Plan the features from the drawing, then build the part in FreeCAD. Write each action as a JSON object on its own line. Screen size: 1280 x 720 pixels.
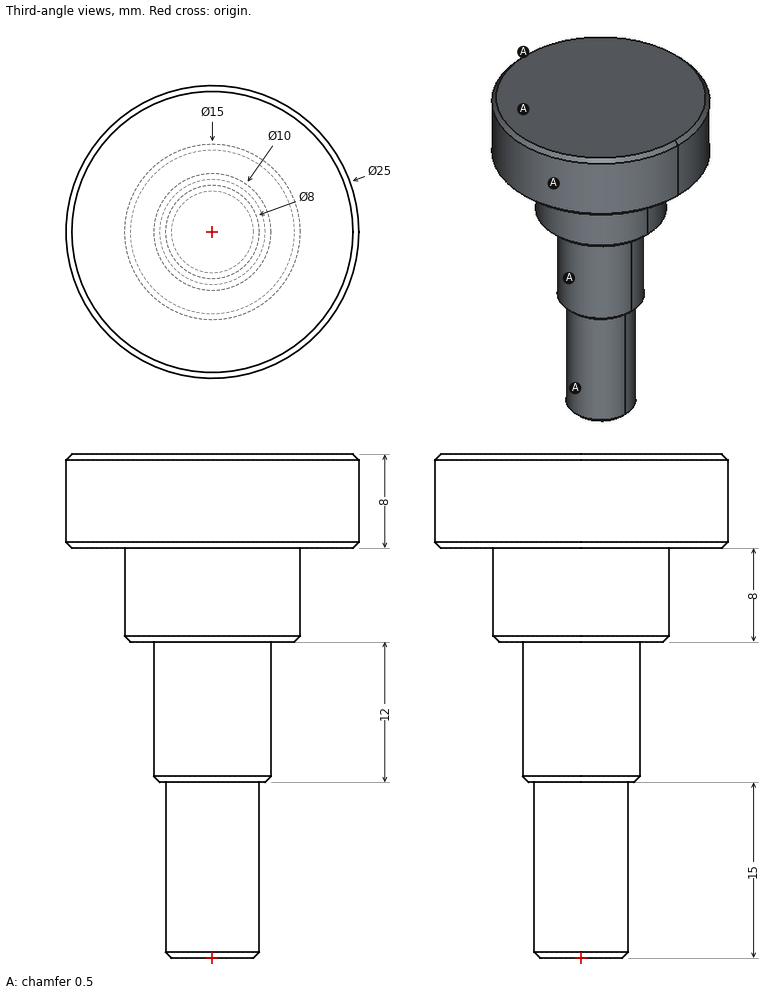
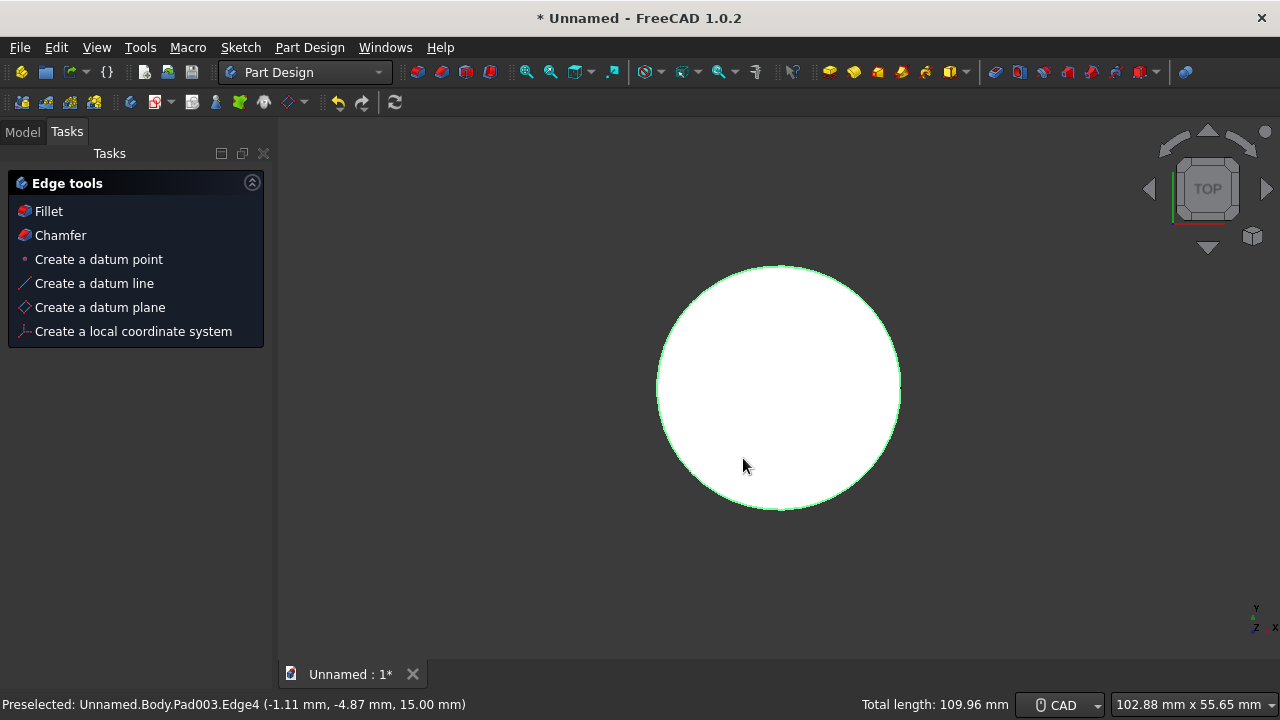
{"action": "key", "text": "1"}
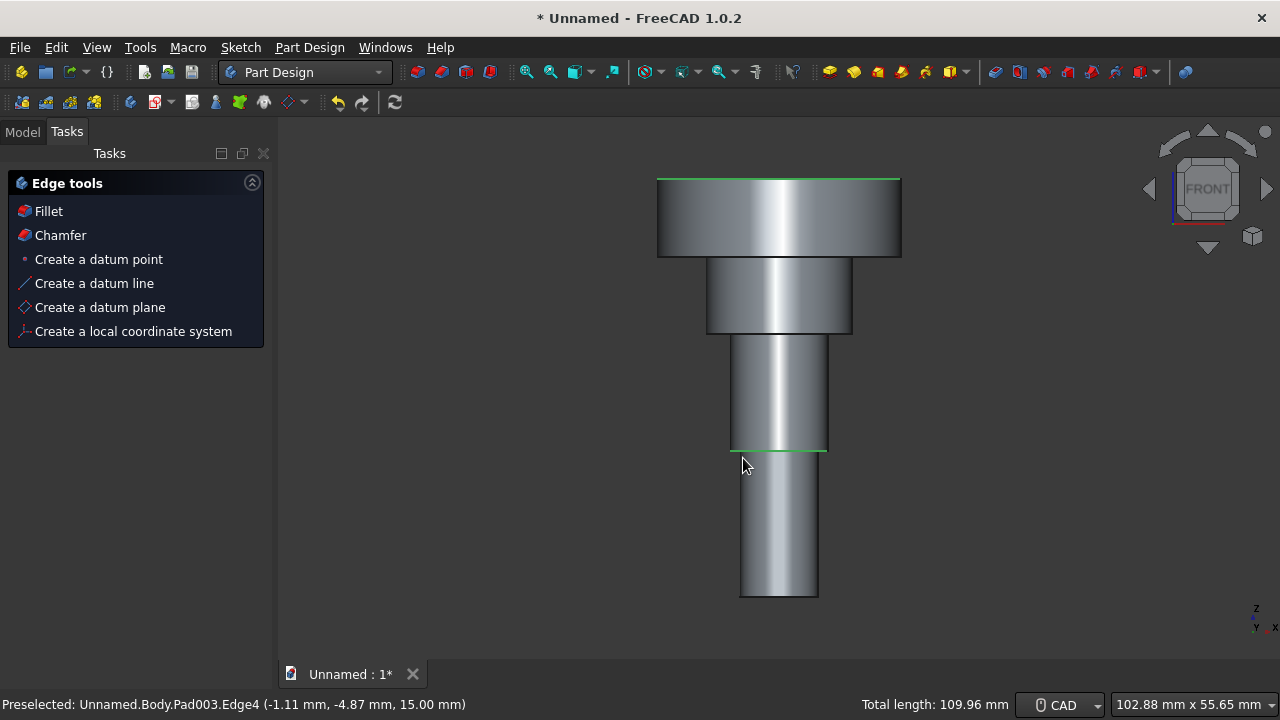
{"action": "left_click", "coordinate": [680, 256], "text": "ctrl"}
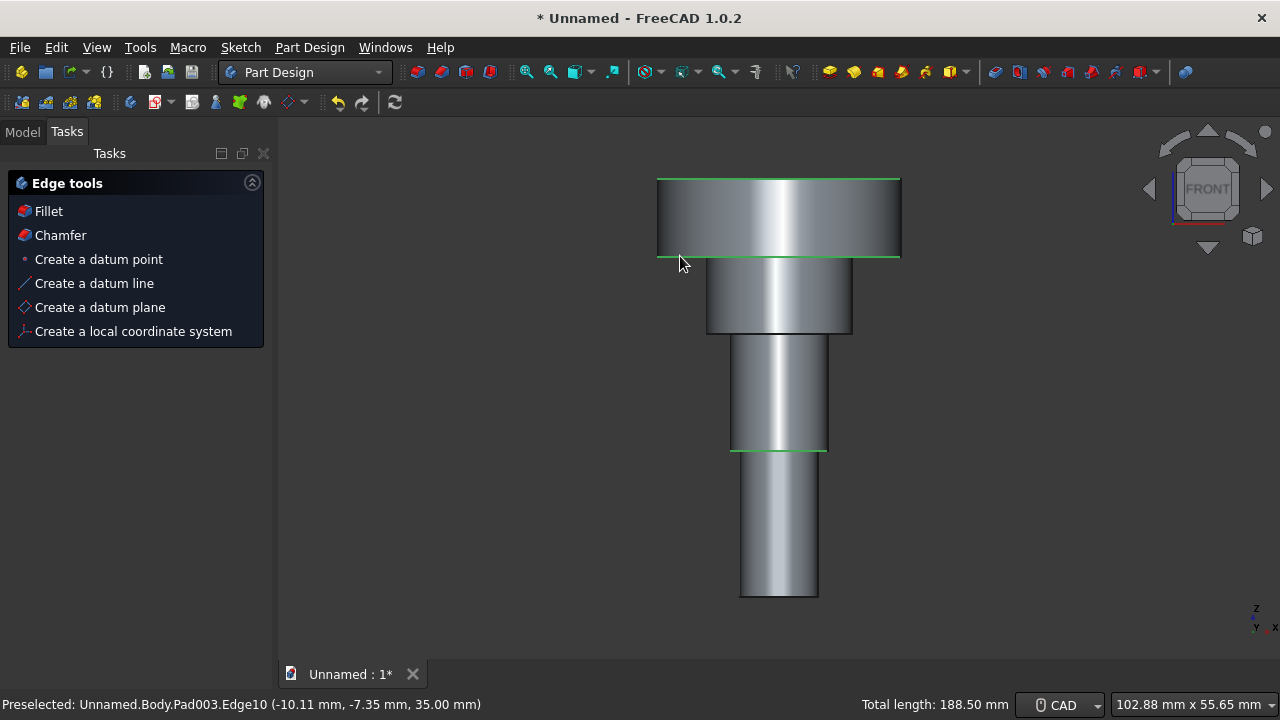
{"action": "left_click", "coordinate": [747, 596], "text": "ctrl"}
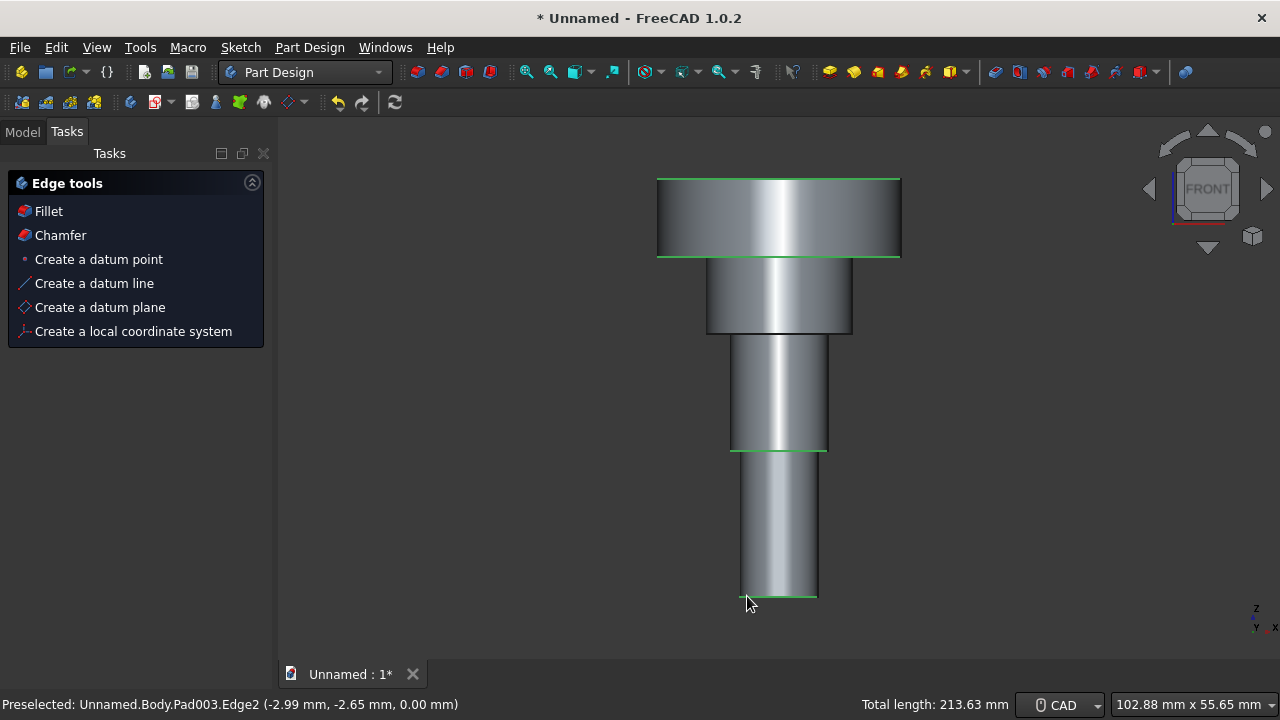
{"action": "left_click", "coordinate": [720, 333], "text": "ctrl"}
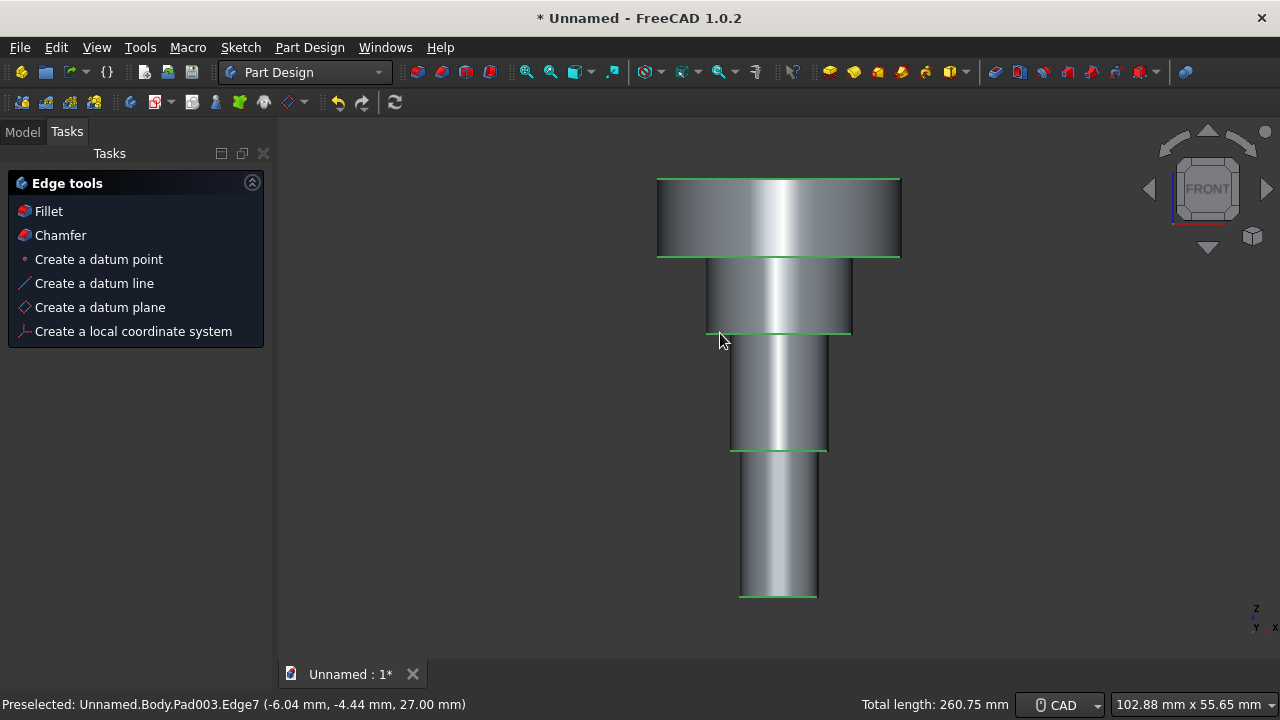
{"action": "left_click", "coordinate": [442, 72]}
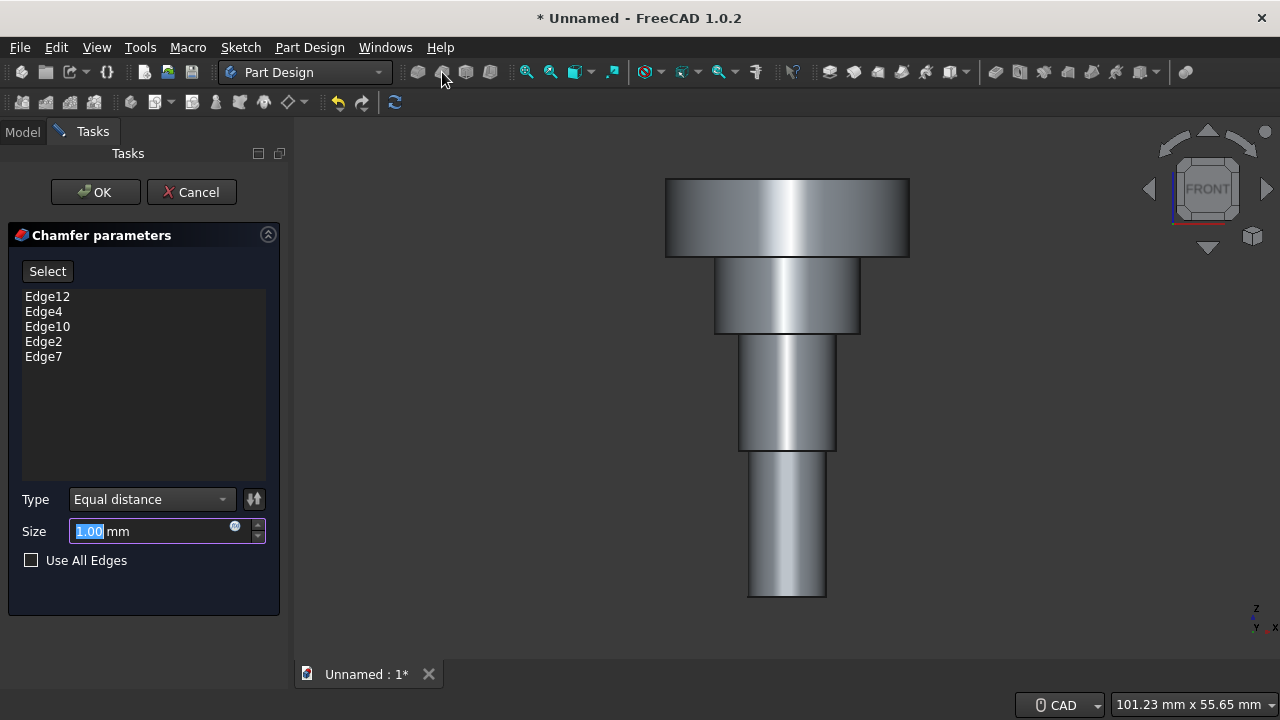
{"action": "type", "text": "0.5"}
{"action": "key", "text": "Tab"}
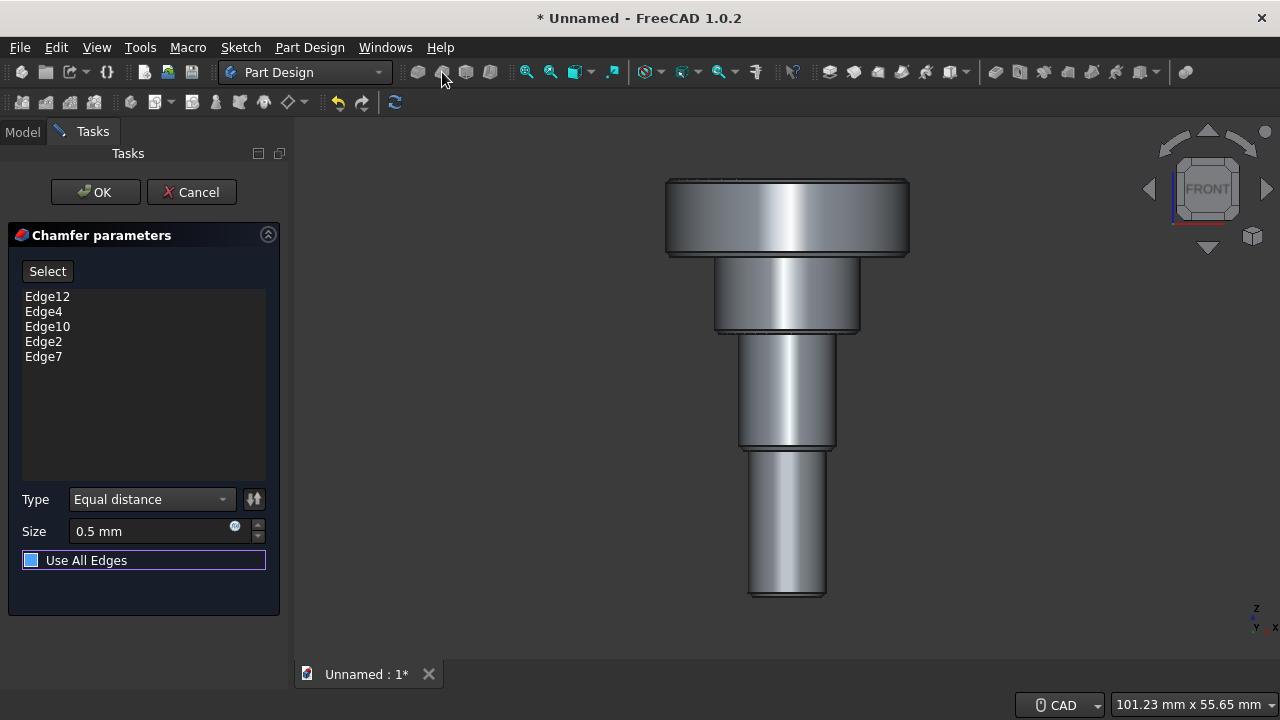
{"action": "left_click", "coordinate": [96, 192]}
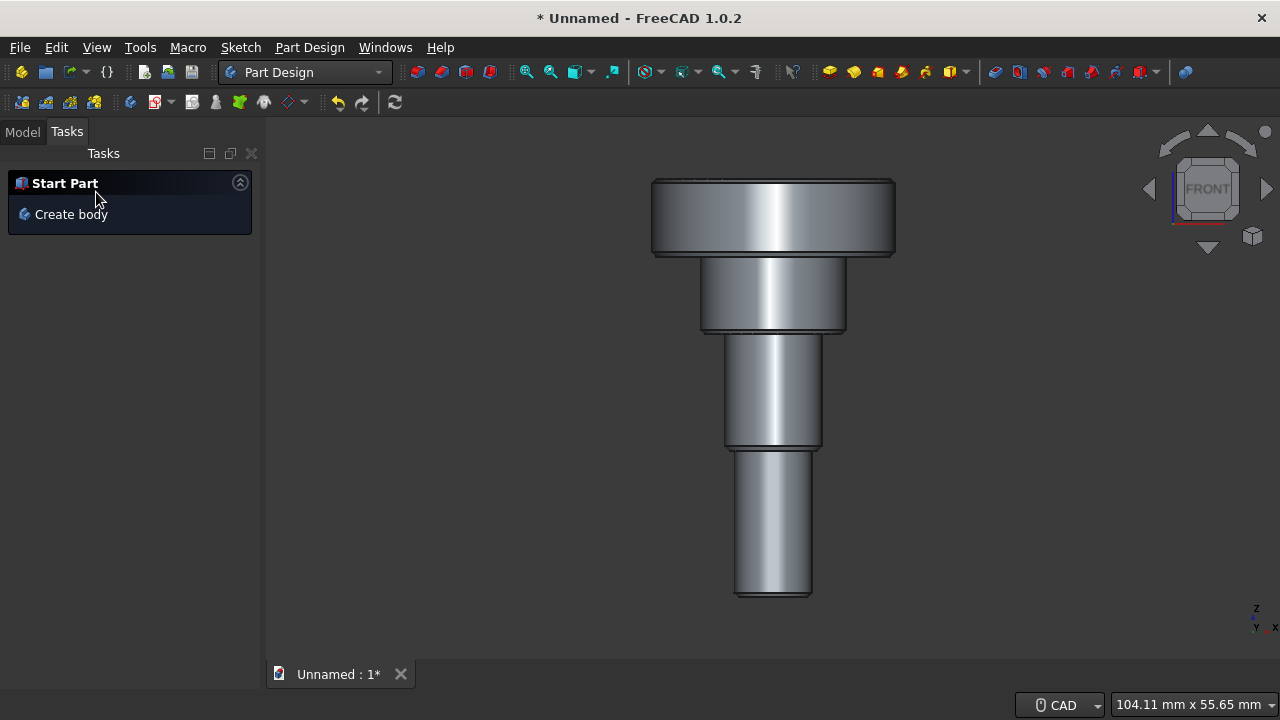
{"action": "key", "text": "0"}